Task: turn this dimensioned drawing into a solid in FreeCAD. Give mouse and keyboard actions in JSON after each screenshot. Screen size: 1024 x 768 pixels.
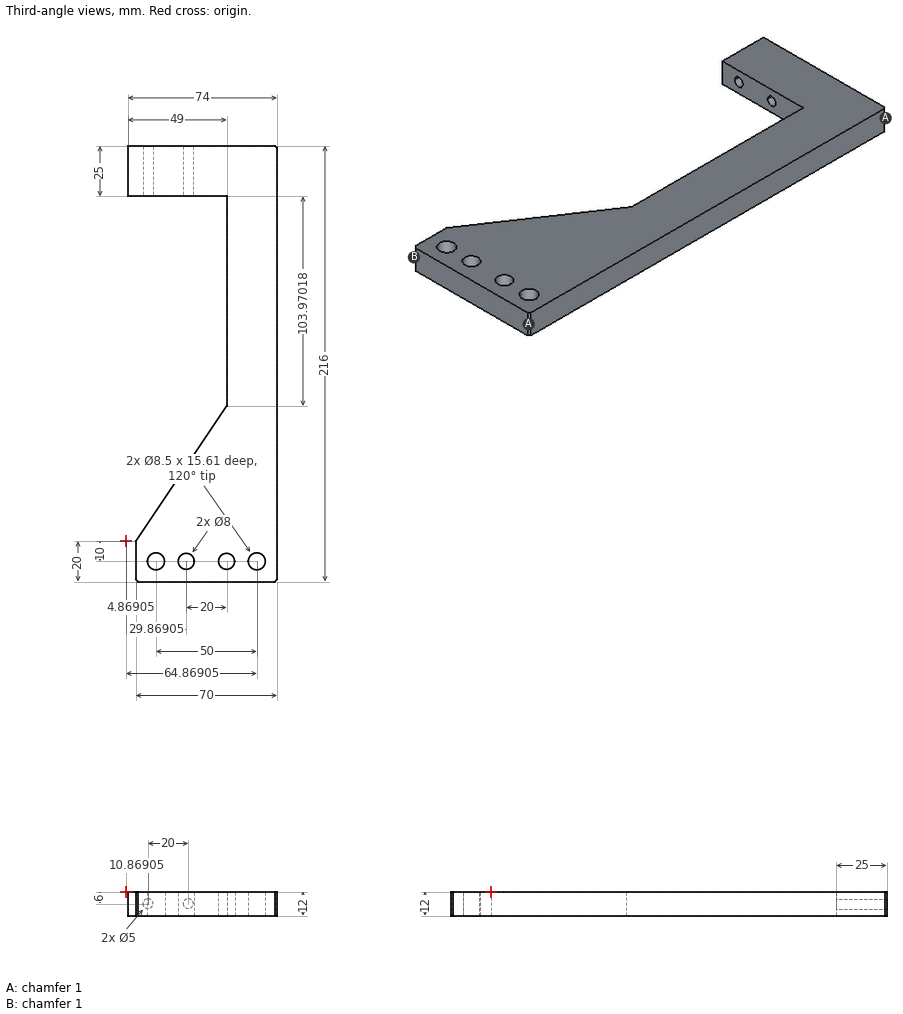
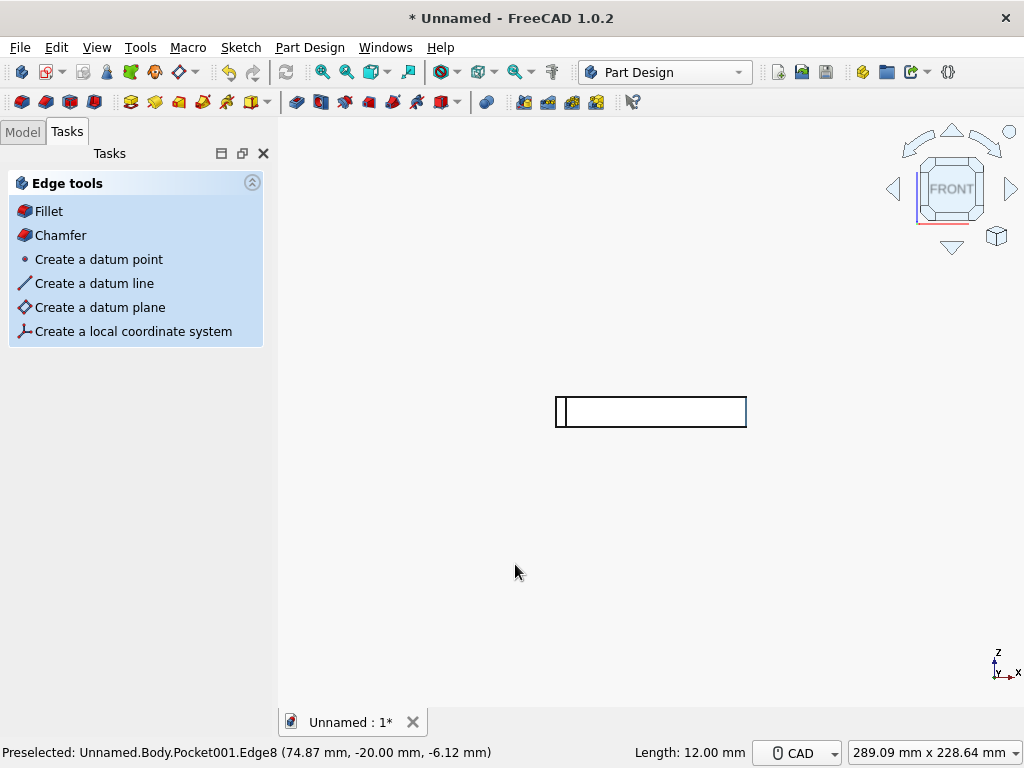
{"action": "key", "text": "v f"}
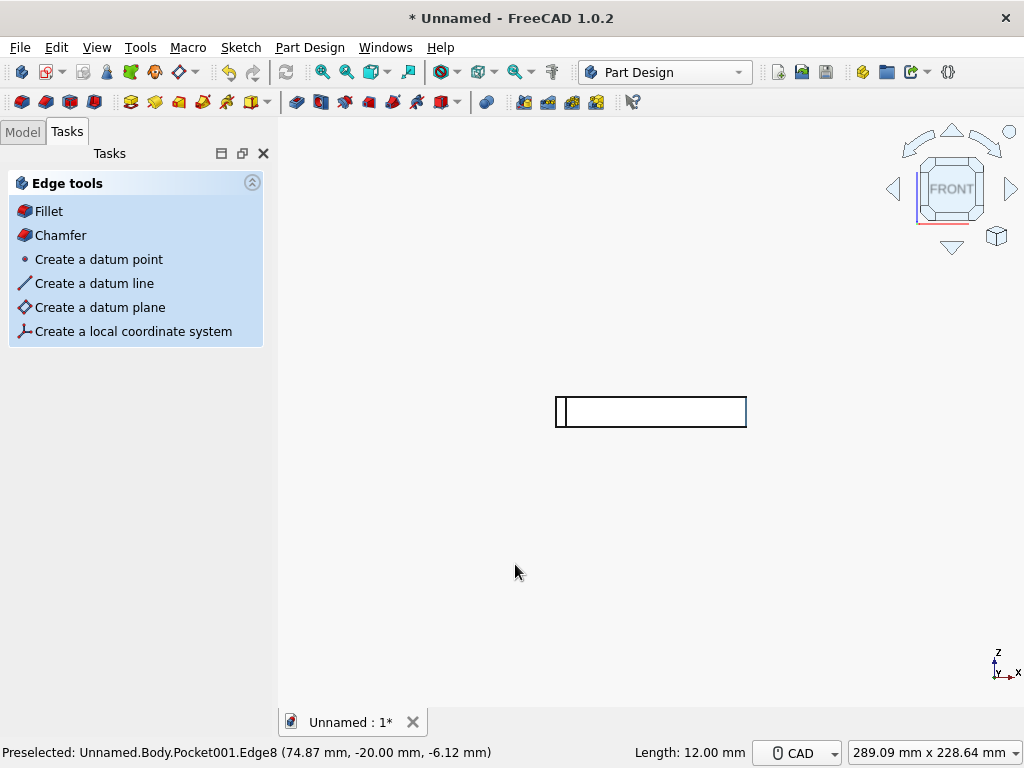
{"action": "key", "text": "3"}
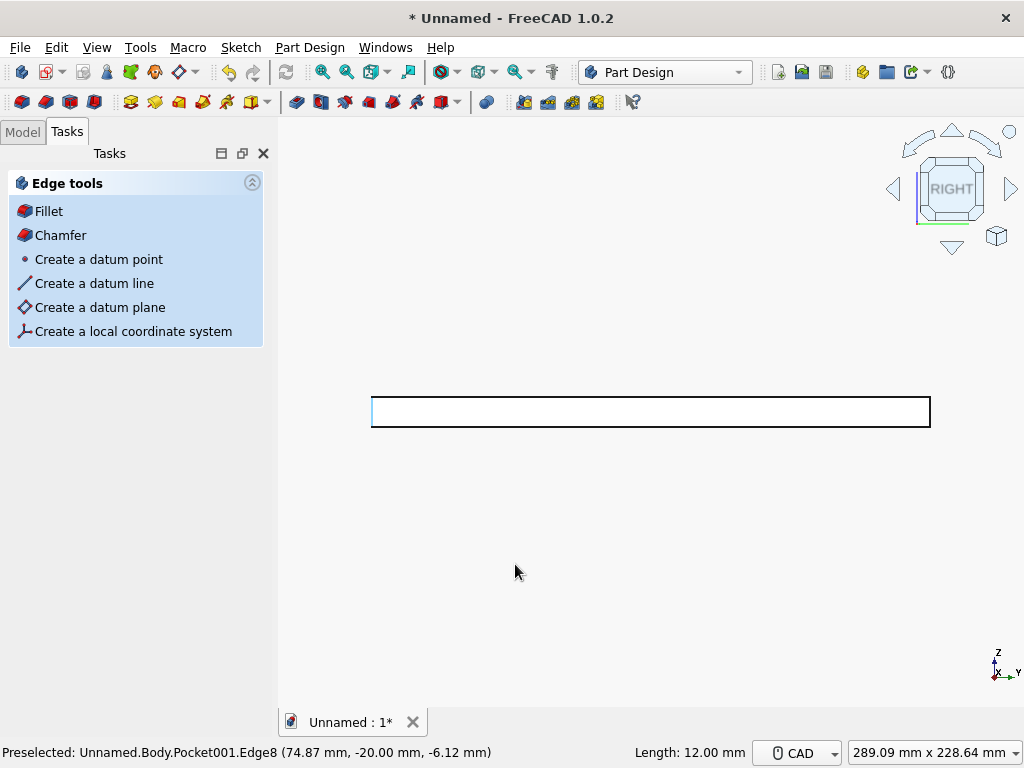
{"action": "left_click", "coordinate": [930, 411], "text": "ctrl"}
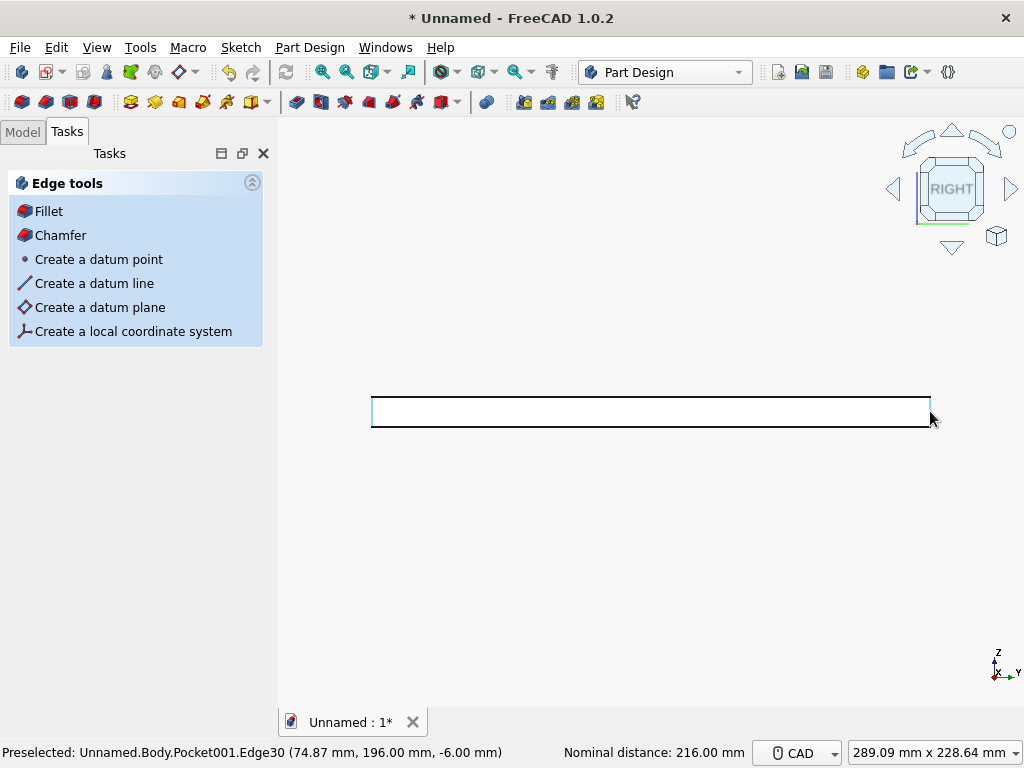
{"action": "left_click", "coordinate": [46, 102]}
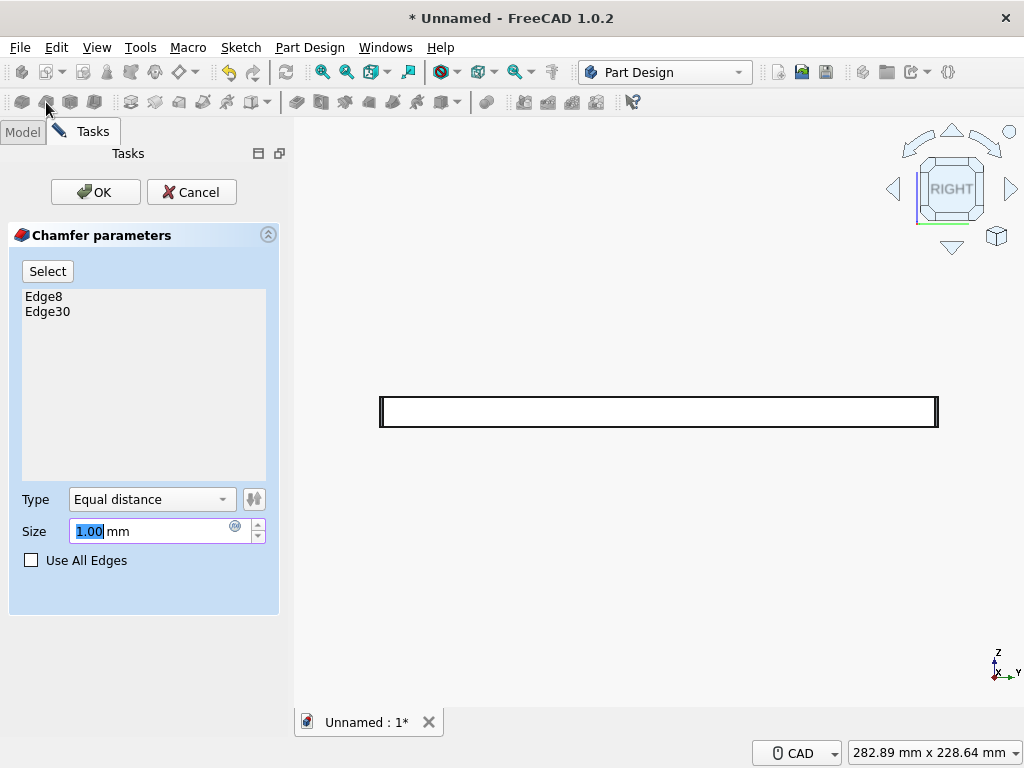
{"action": "type", "text": "1"}
{"action": "key", "text": "Tab"}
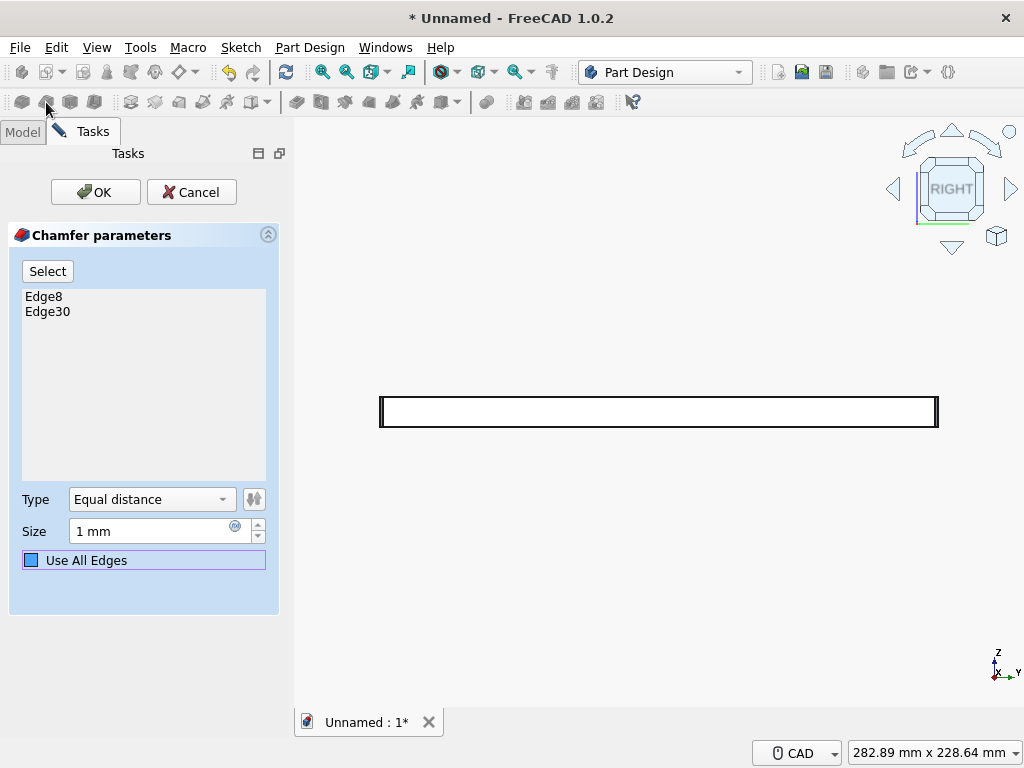
{"action": "left_click", "coordinate": [96, 192]}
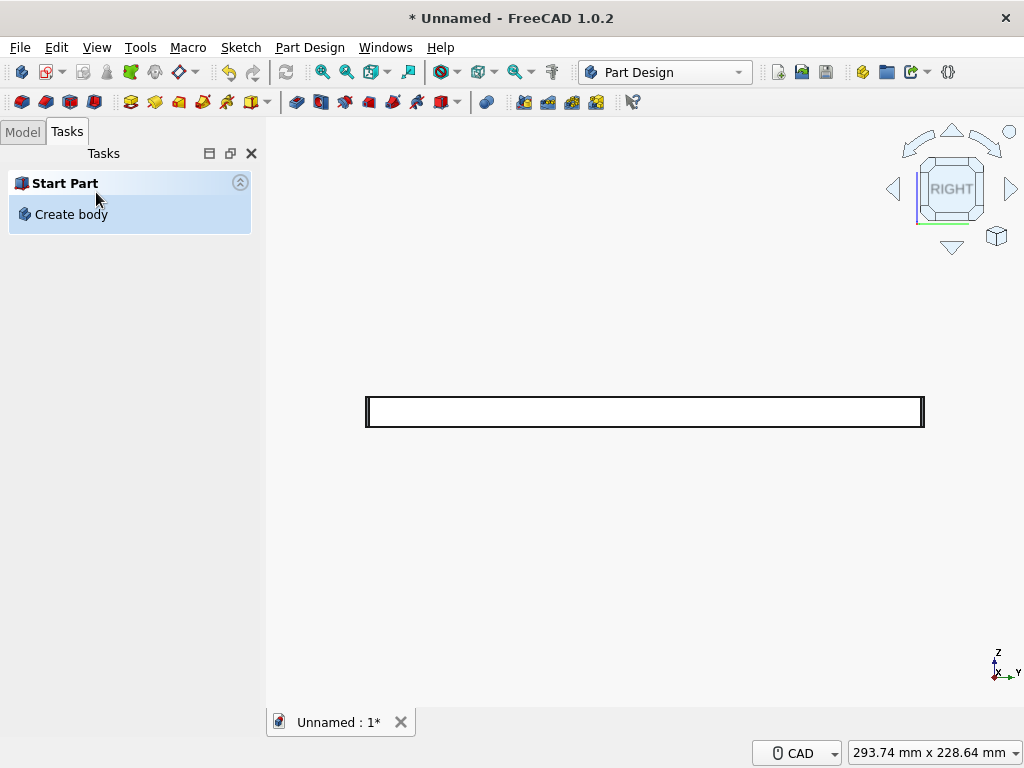
{"action": "key", "text": "0"}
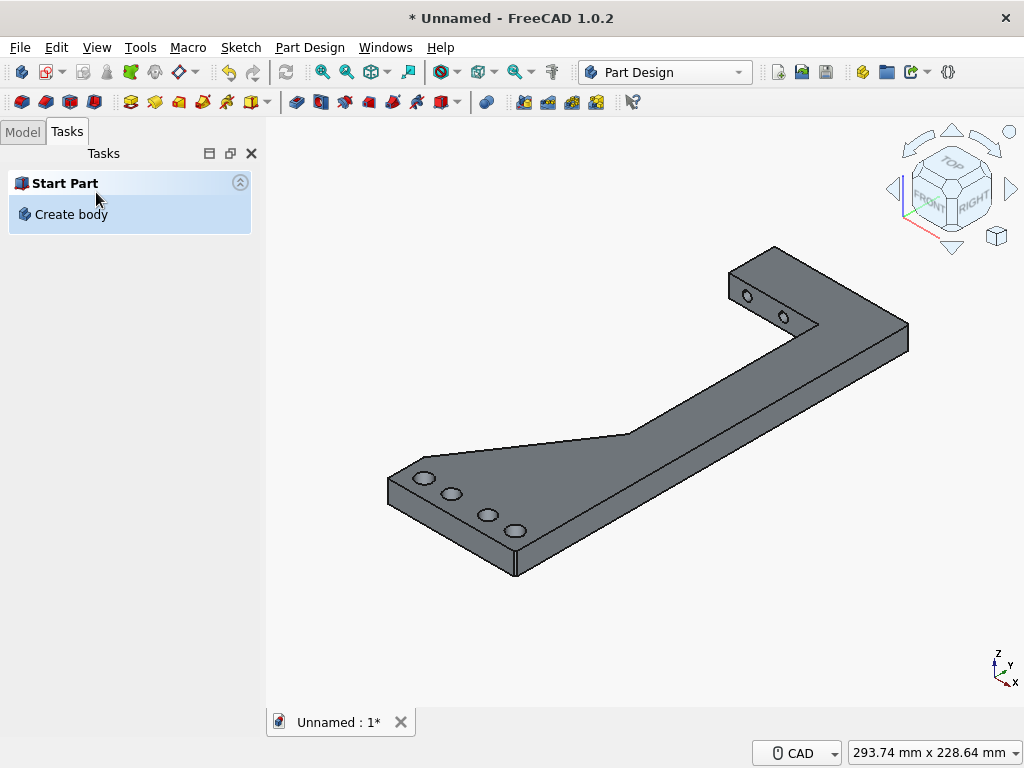
{"action": "key", "text": "2"}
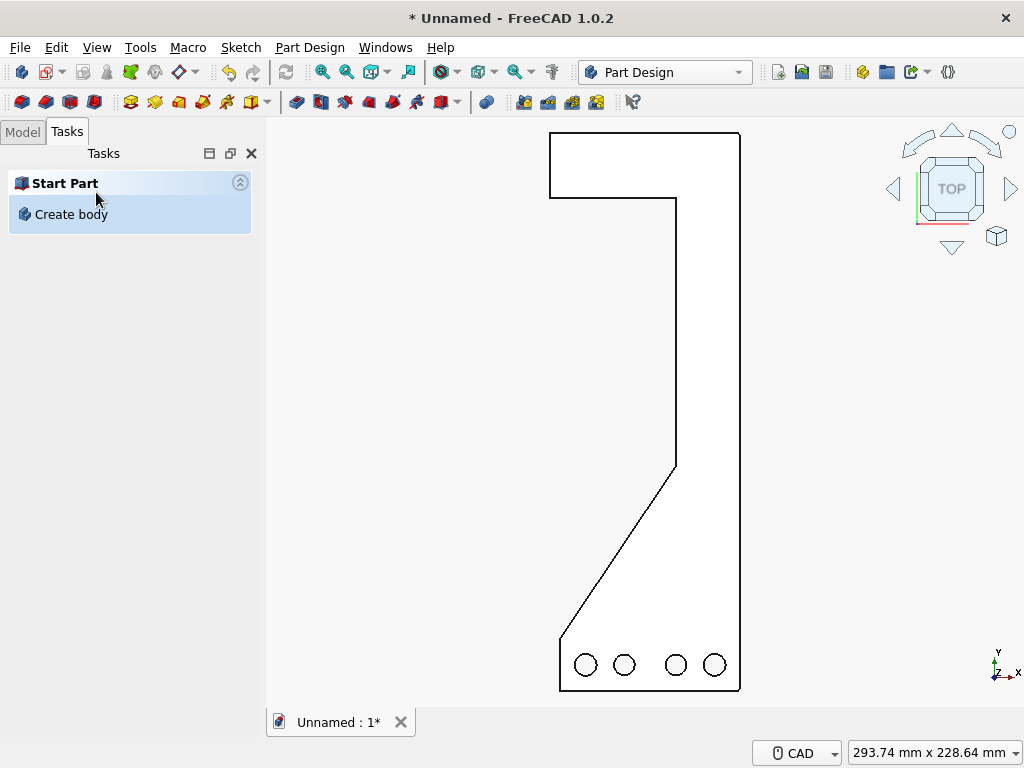
{"action": "key", "text": "1"}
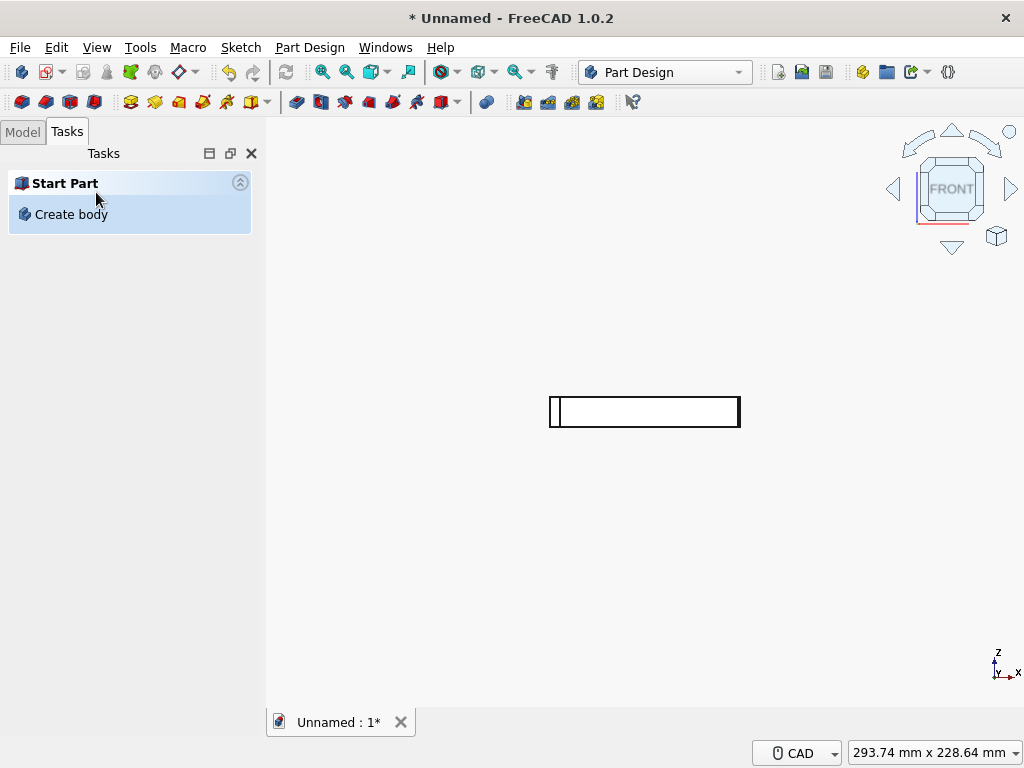
{"action": "key", "text": "v f"}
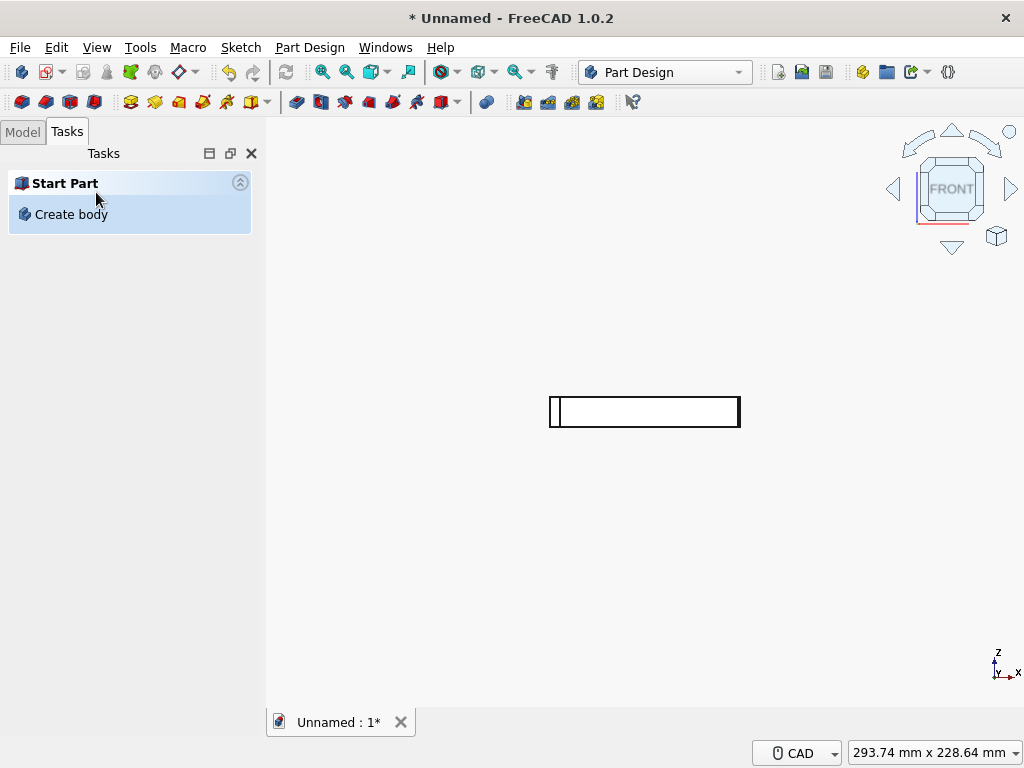
{"action": "left_click", "coordinate": [560, 411]}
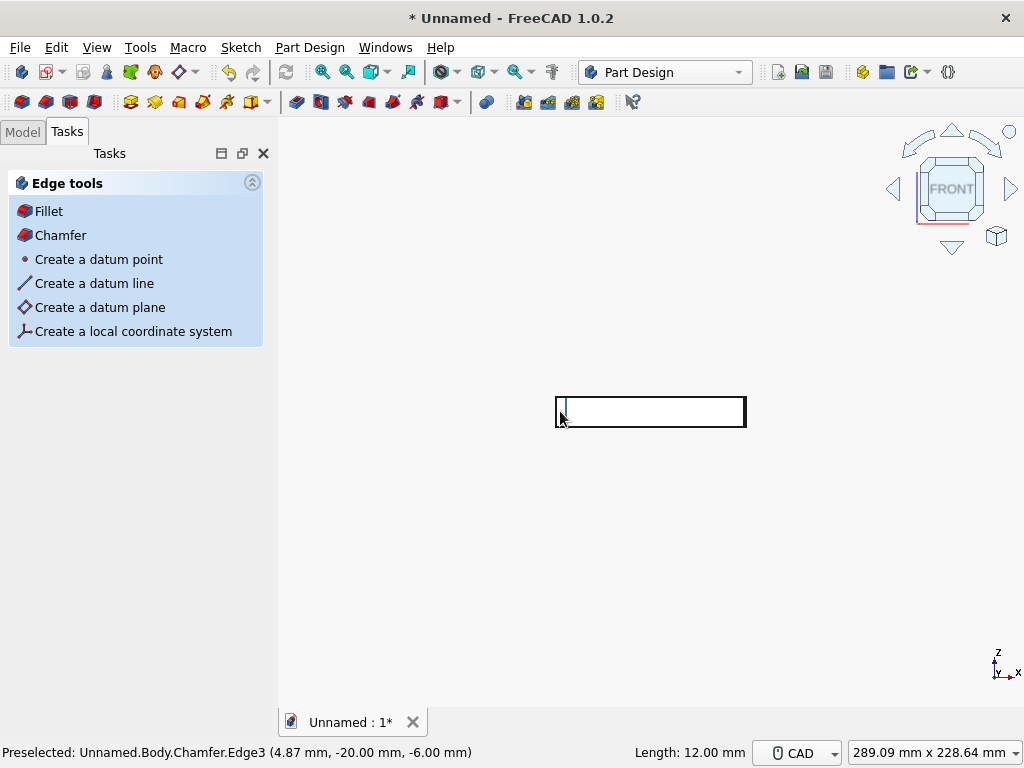
{"action": "left_click", "coordinate": [46, 102]}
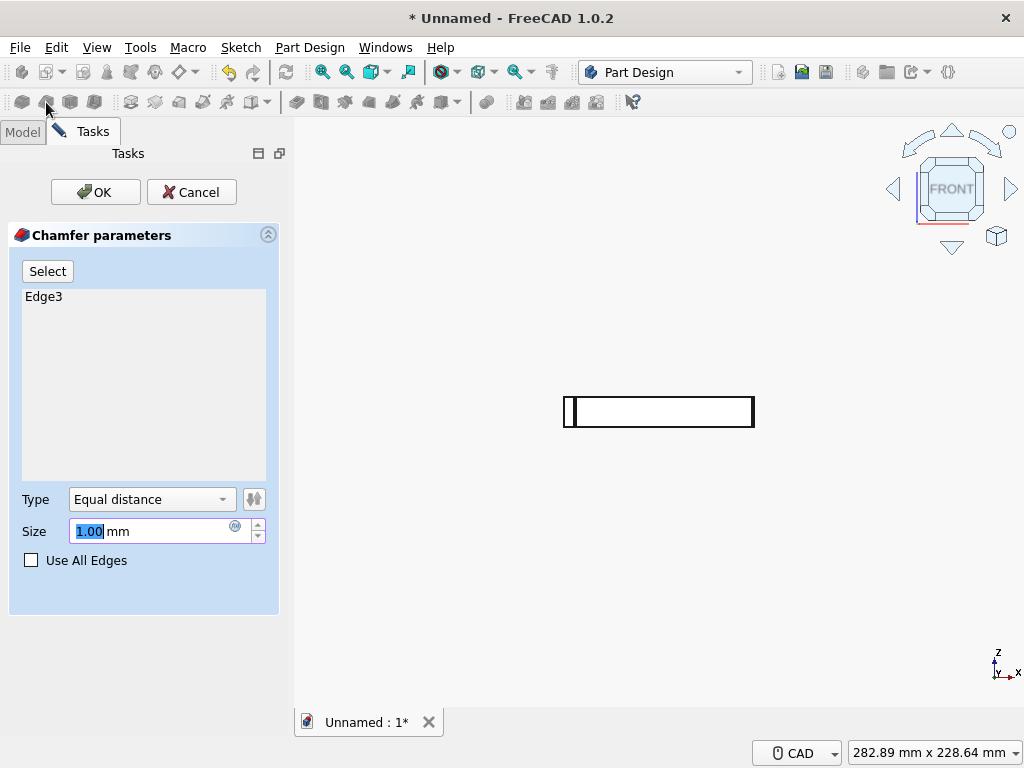
{"action": "type", "text": "1"}
{"action": "key", "text": "Tab"}